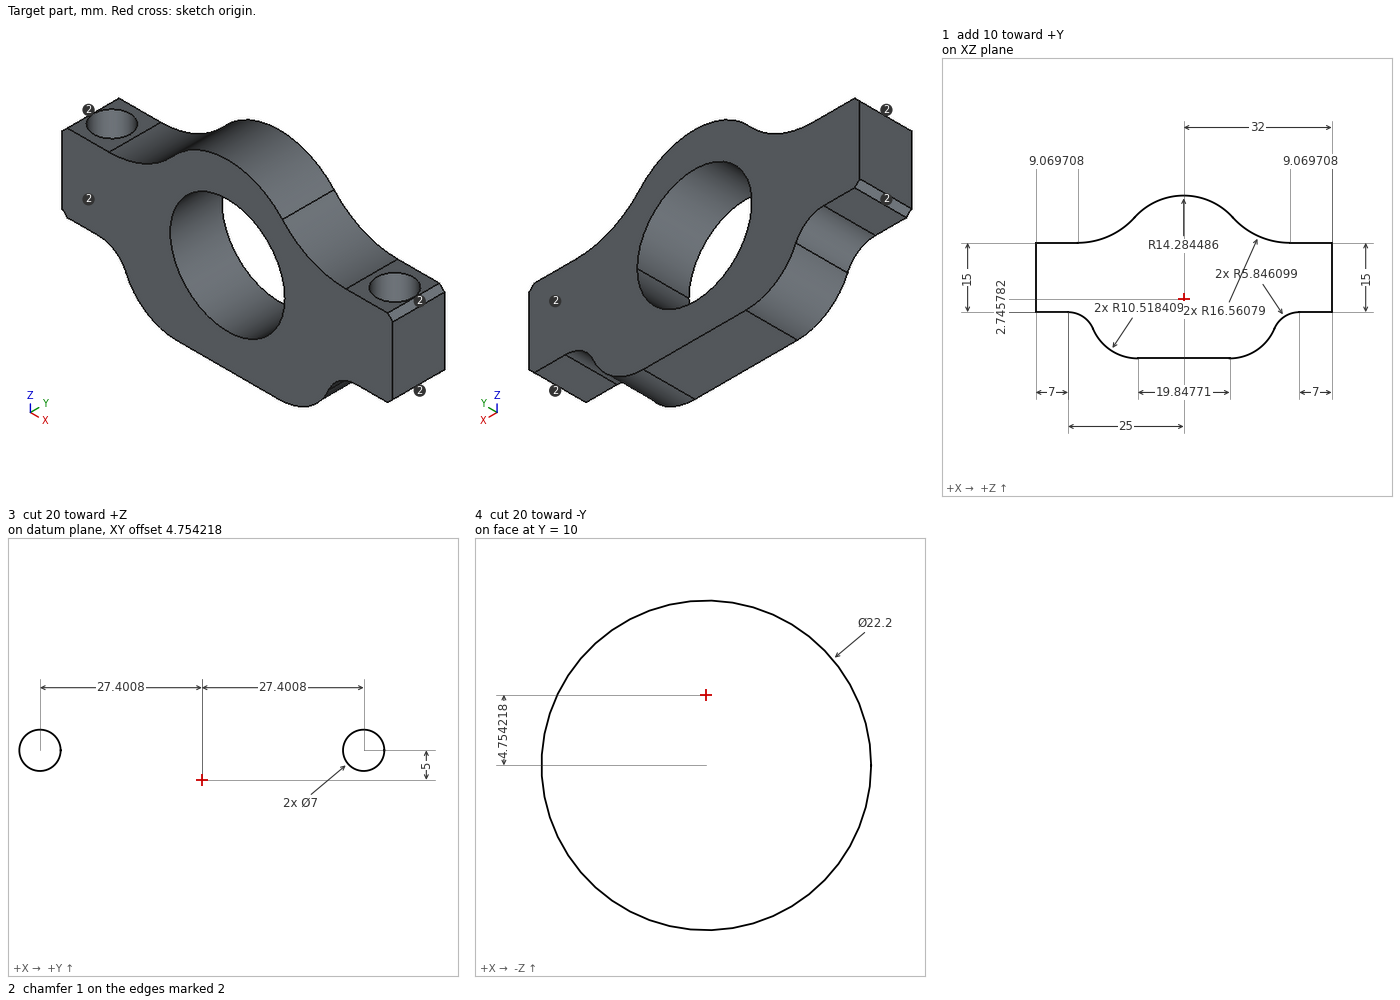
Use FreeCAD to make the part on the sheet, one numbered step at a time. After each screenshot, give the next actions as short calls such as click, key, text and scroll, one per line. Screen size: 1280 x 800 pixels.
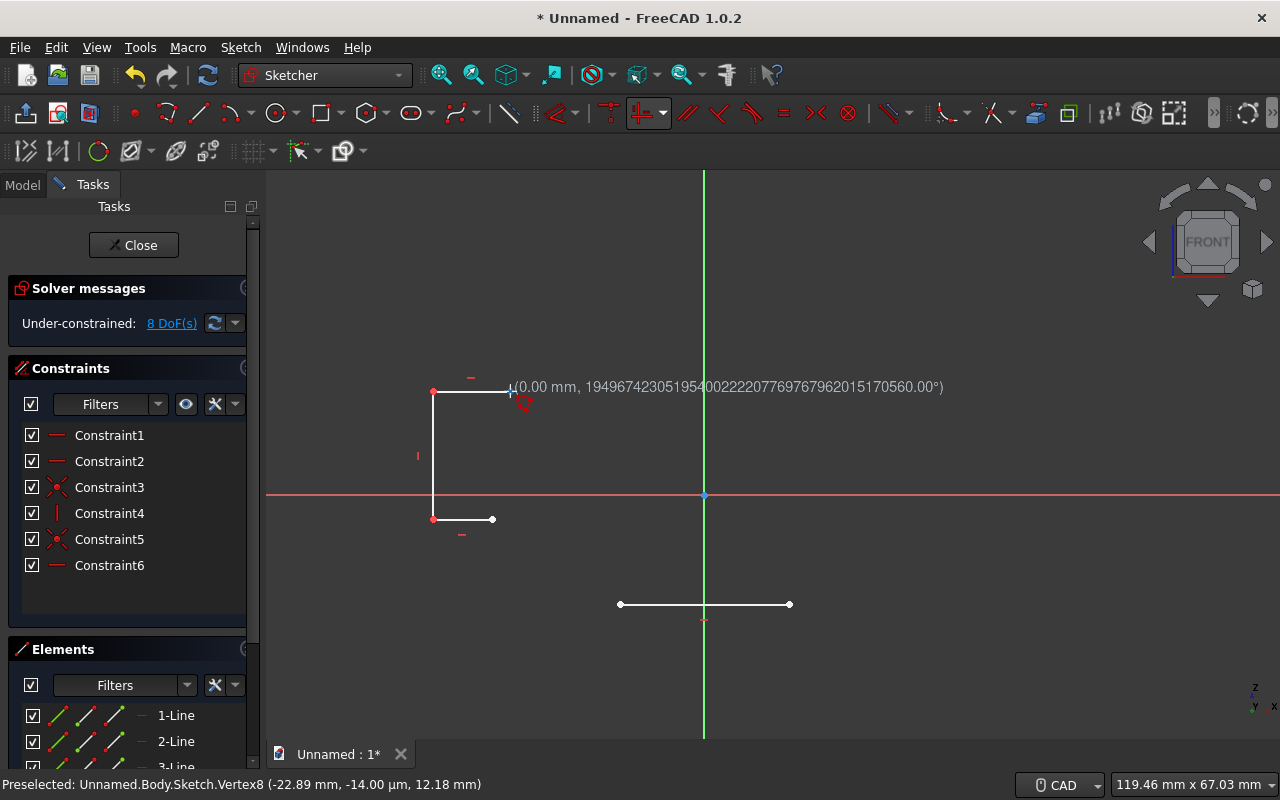
click(899, 391)
click(976, 391)
click(976, 519)
click(917, 519)
right_click(917, 519)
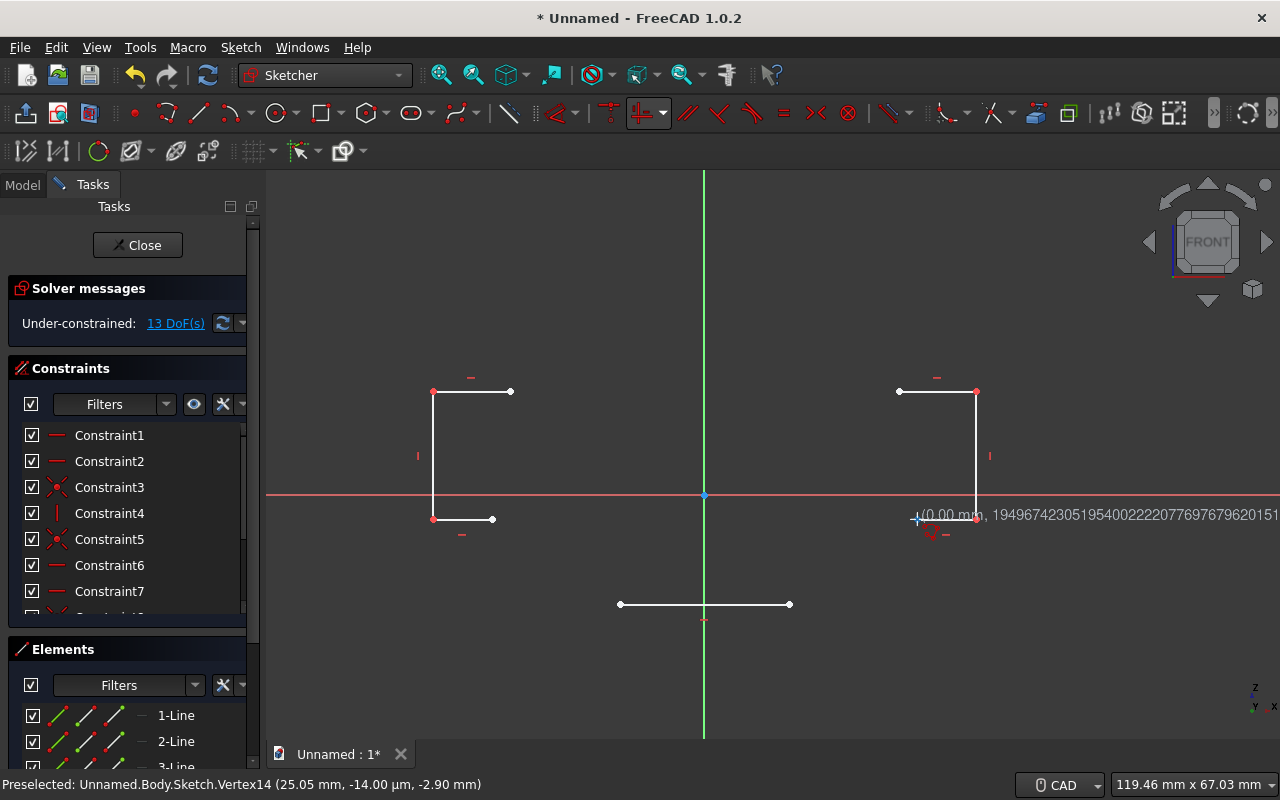
click(254, 114)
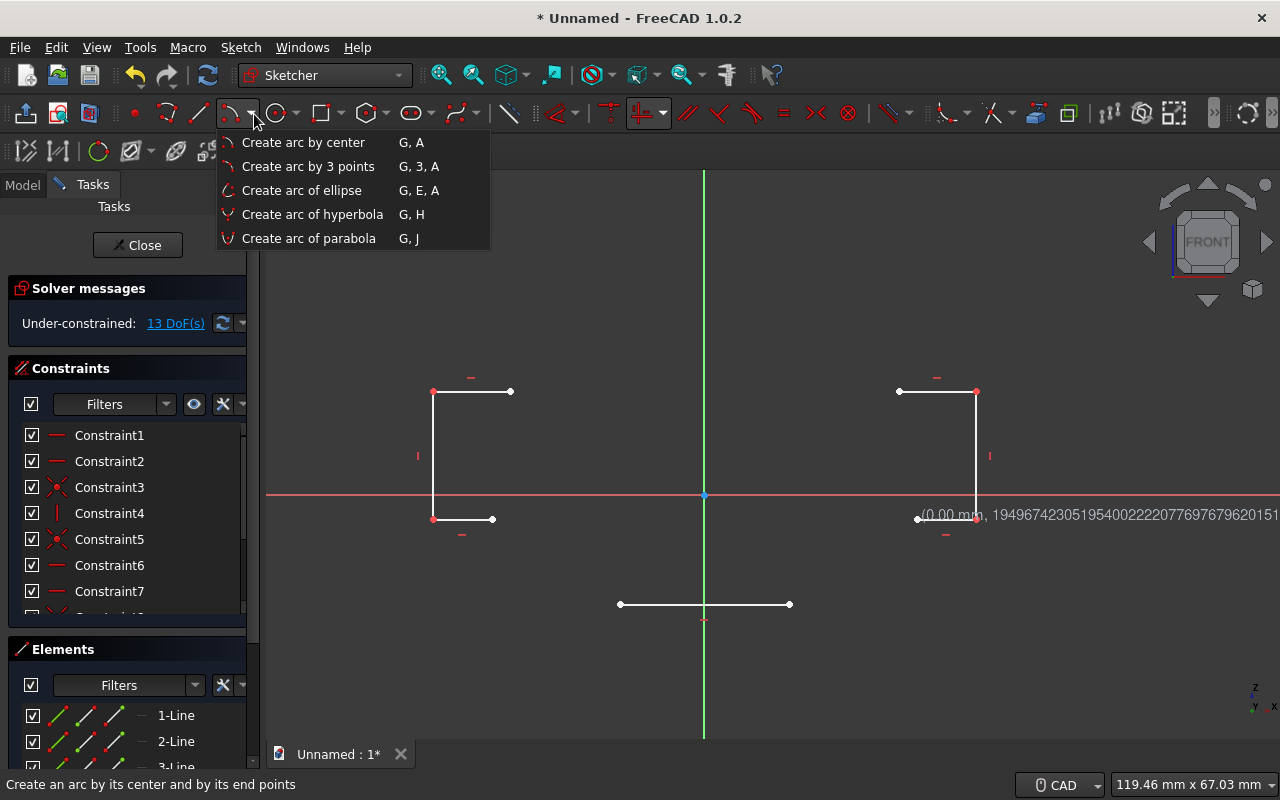
click(354, 166)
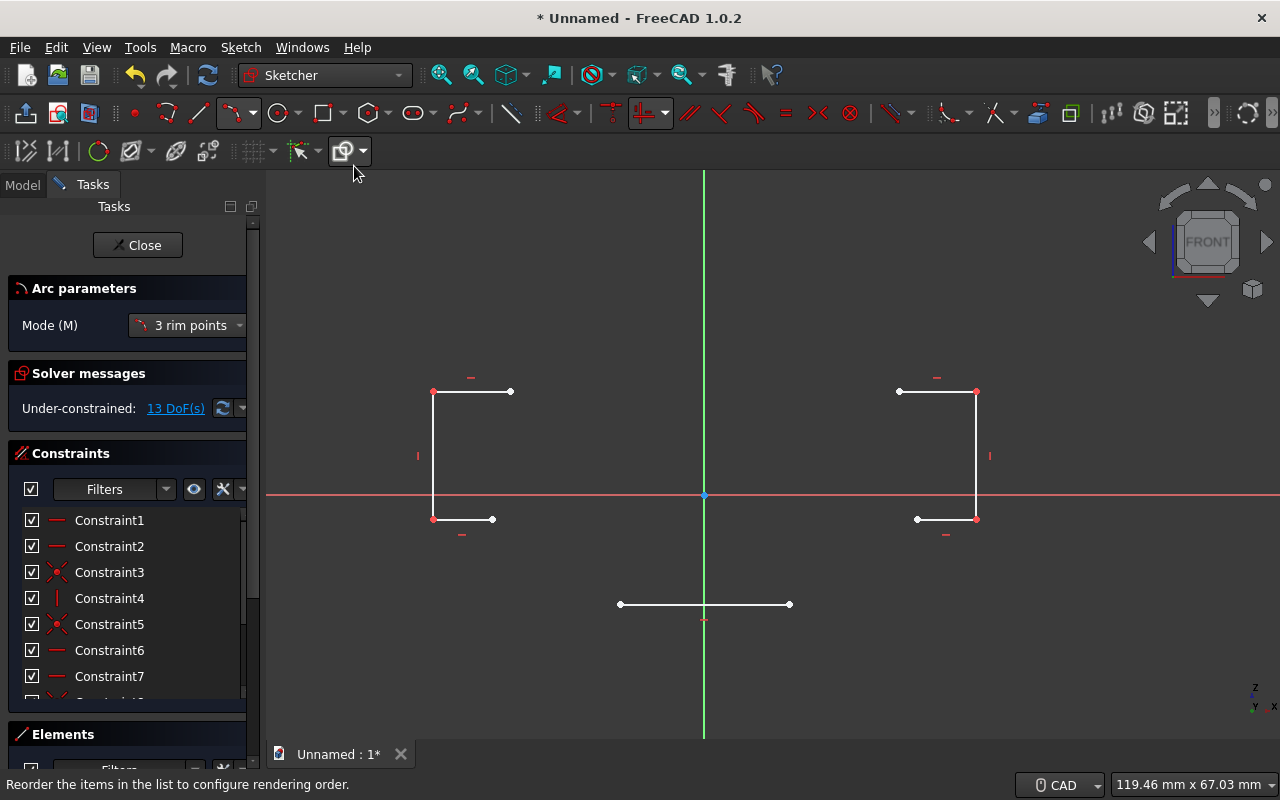
click(620, 605)
click(538, 549)
click(571, 589)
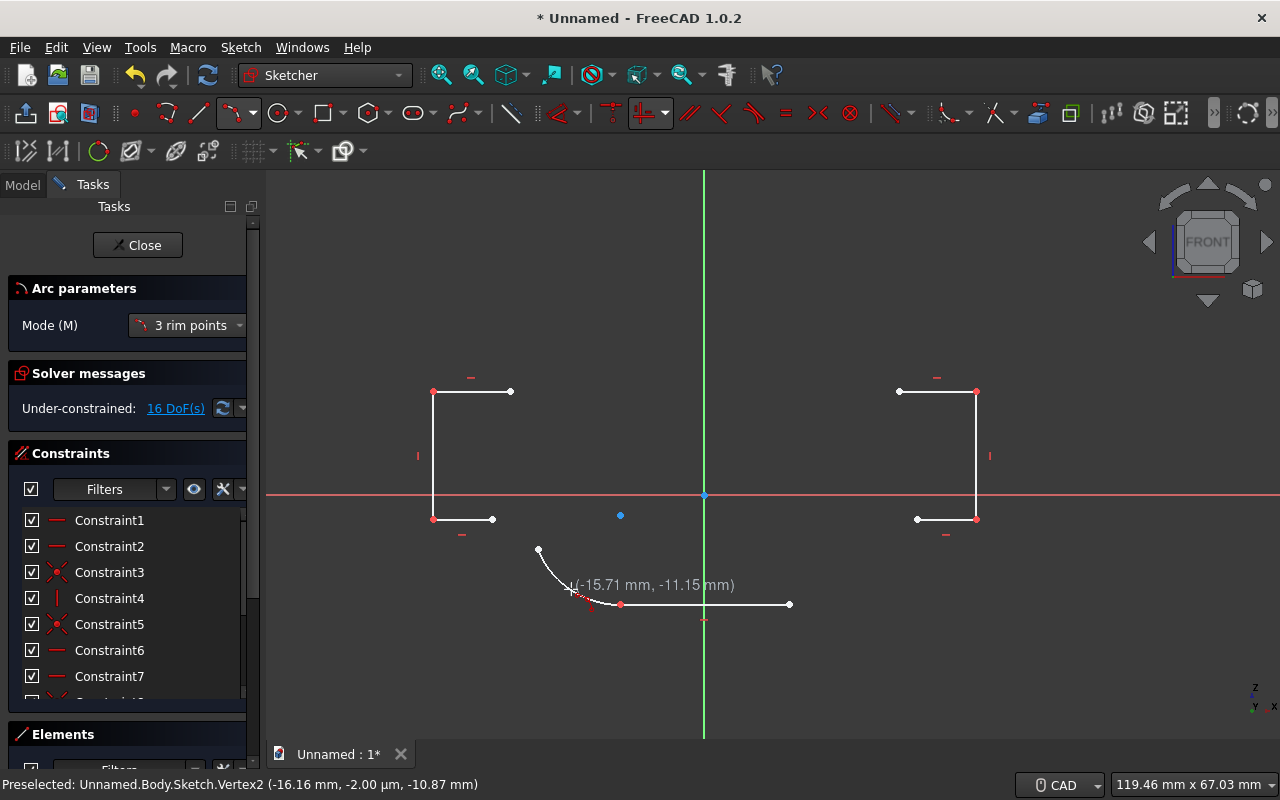
click(538, 550)
click(492, 520)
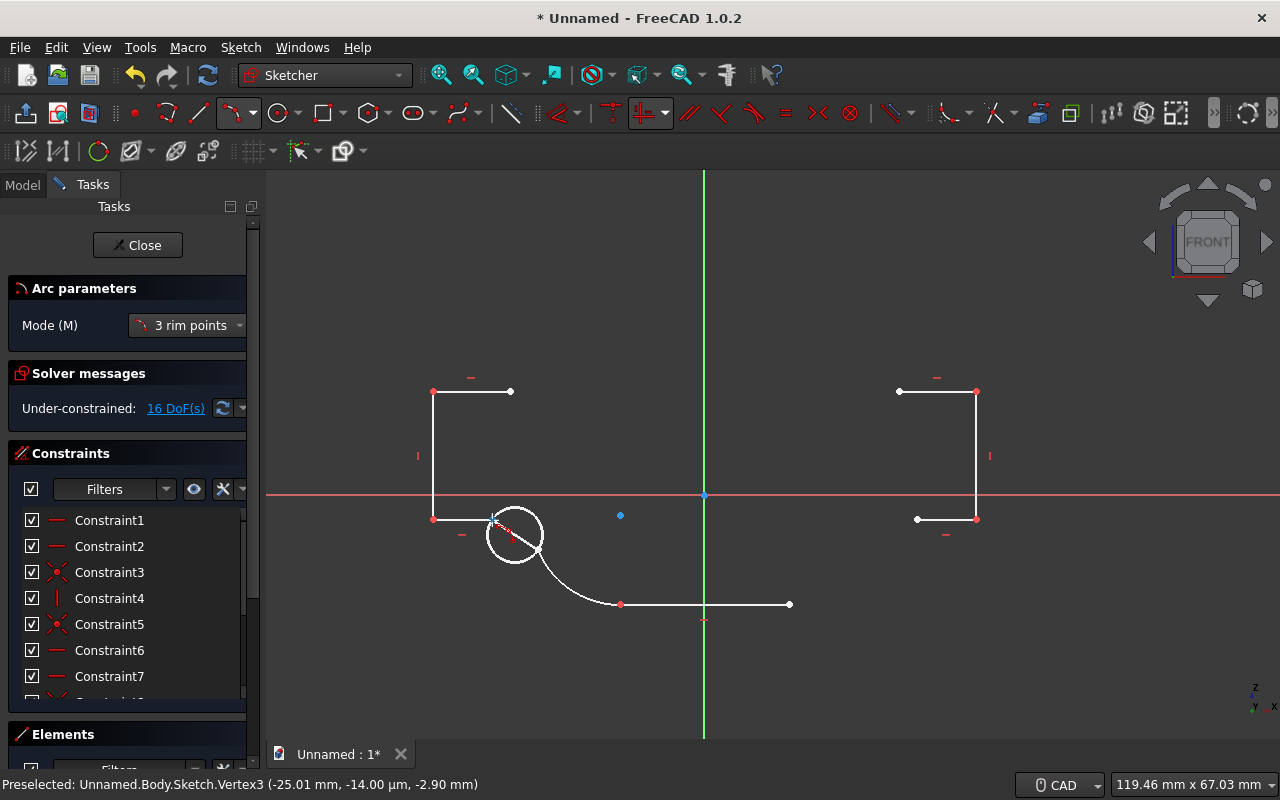
scroll(520, 527, up, 4)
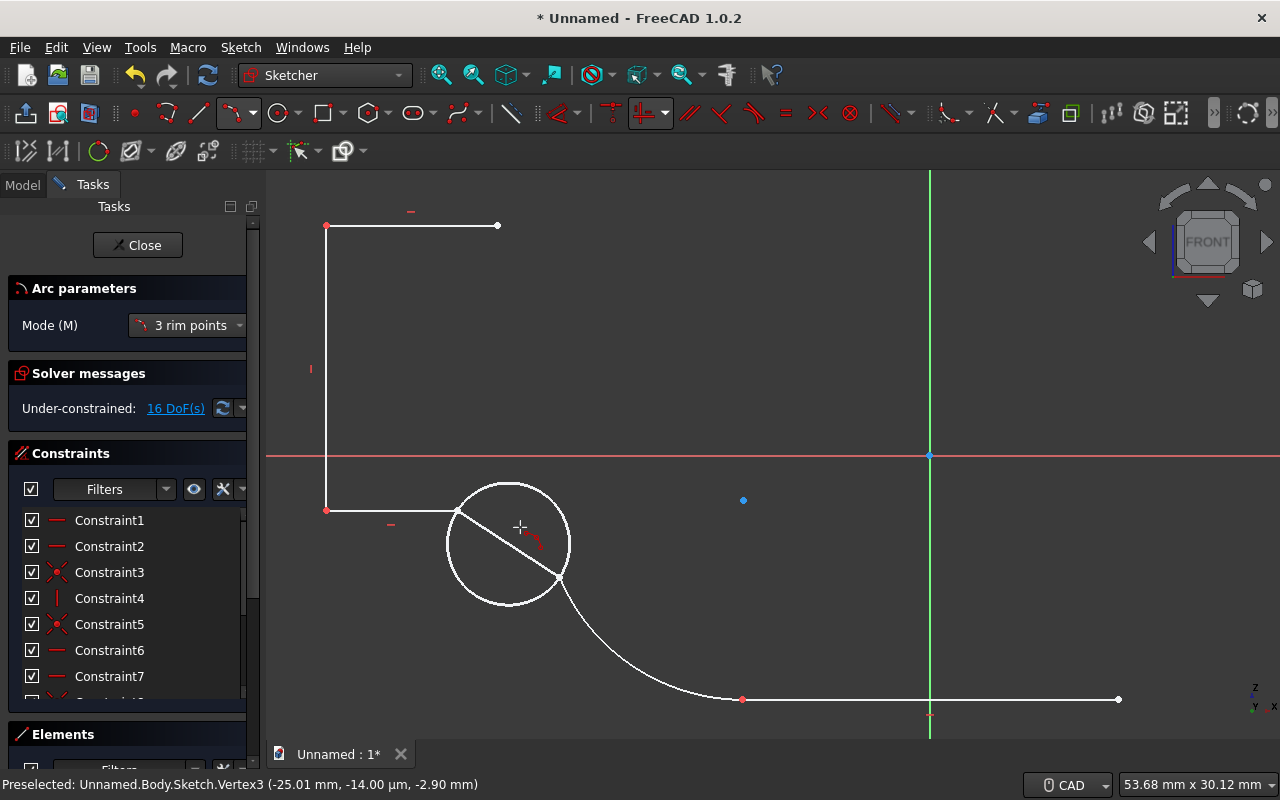
click(519, 526)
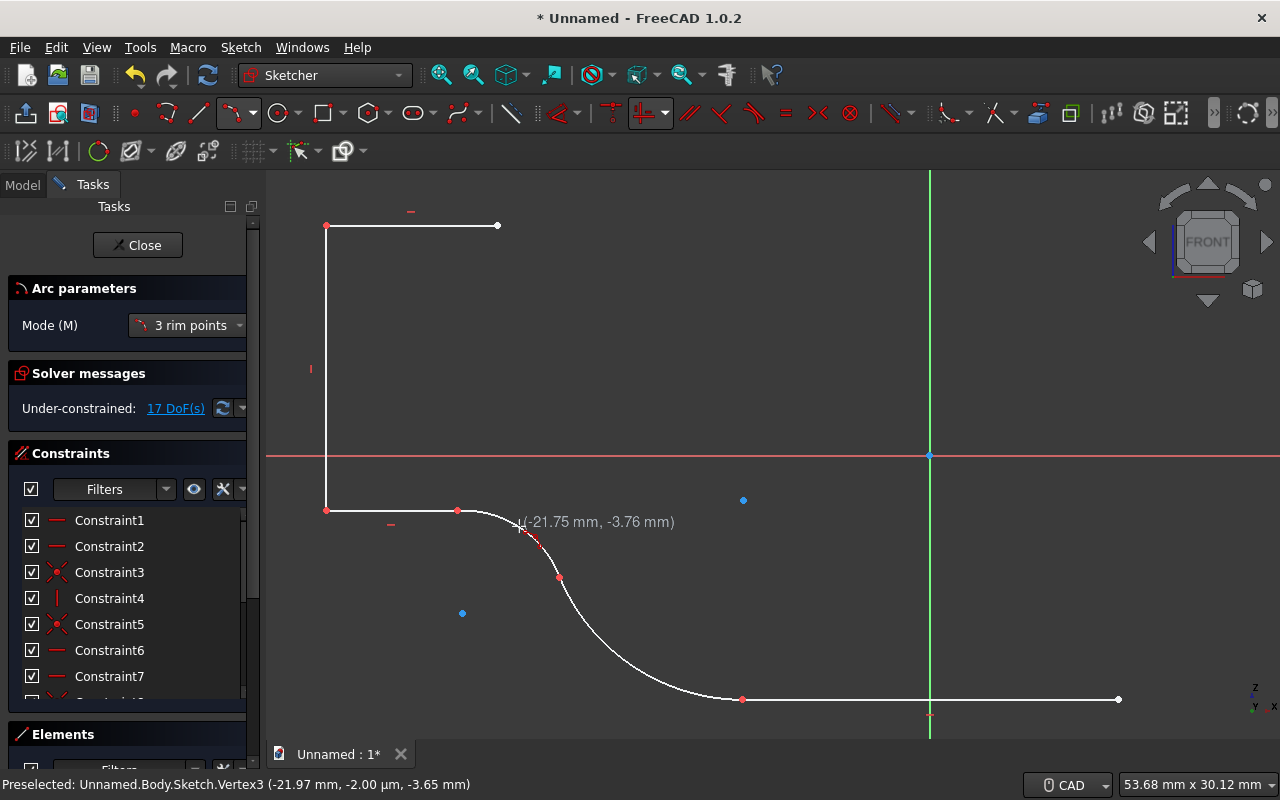
click(497, 226)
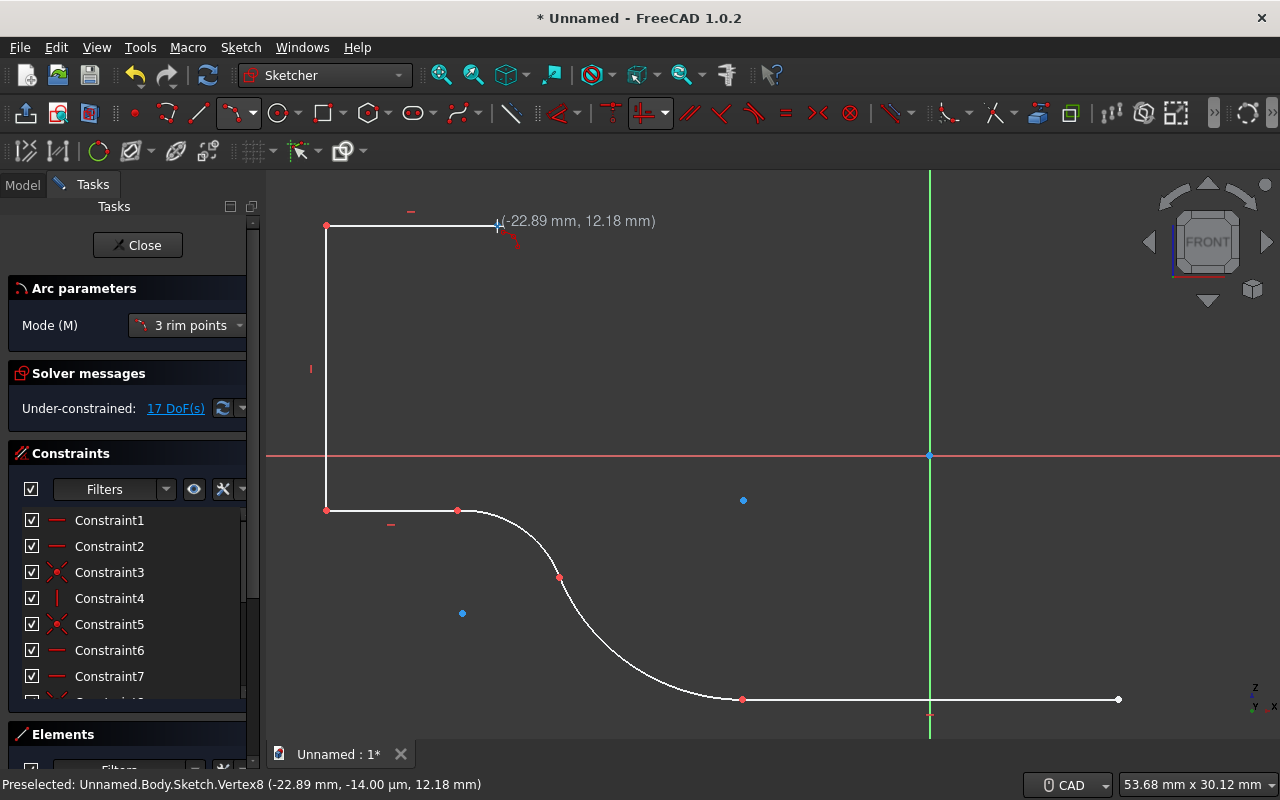
scroll(521, 528, down, 4)